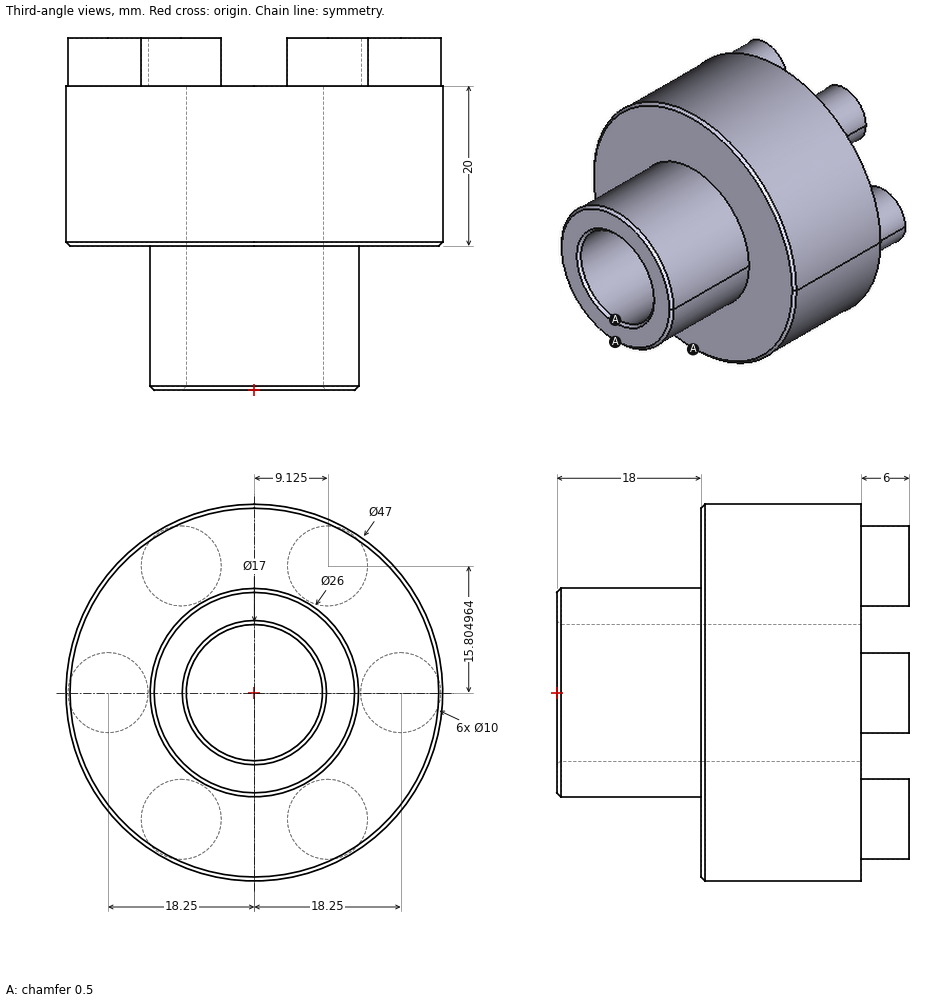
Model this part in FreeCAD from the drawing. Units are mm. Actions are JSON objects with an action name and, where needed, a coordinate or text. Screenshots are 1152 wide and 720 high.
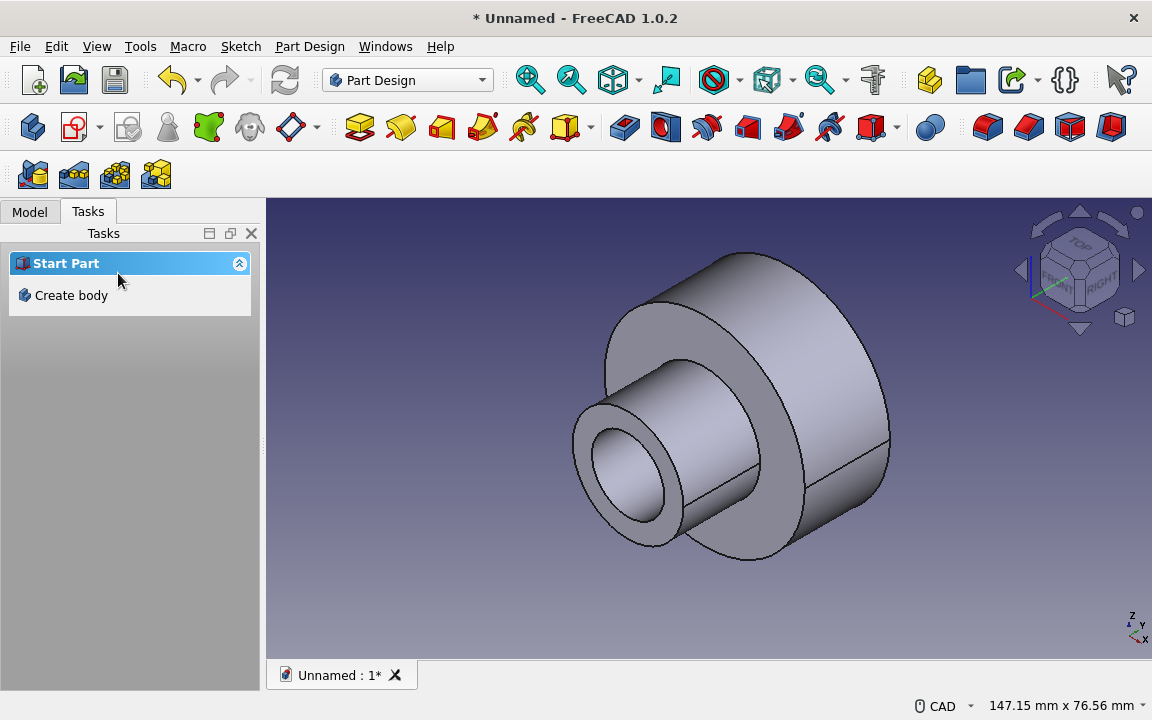
{"action": "key", "text": "4"}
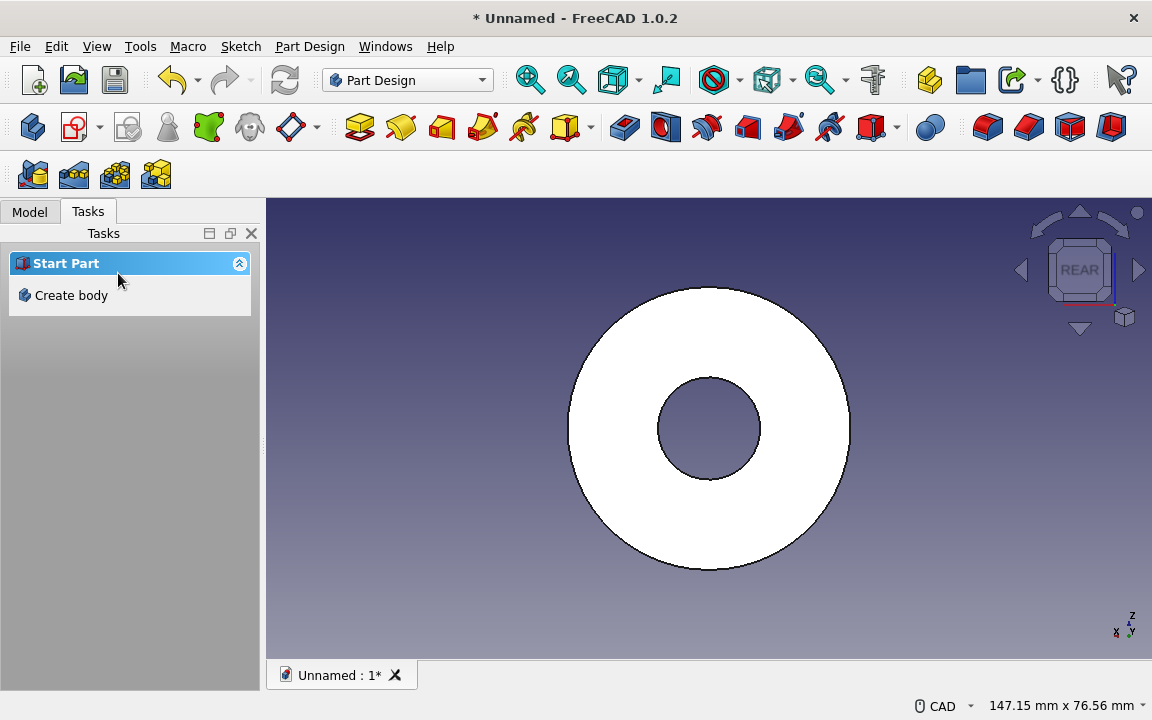
{"action": "left_click", "coordinate": [749, 347]}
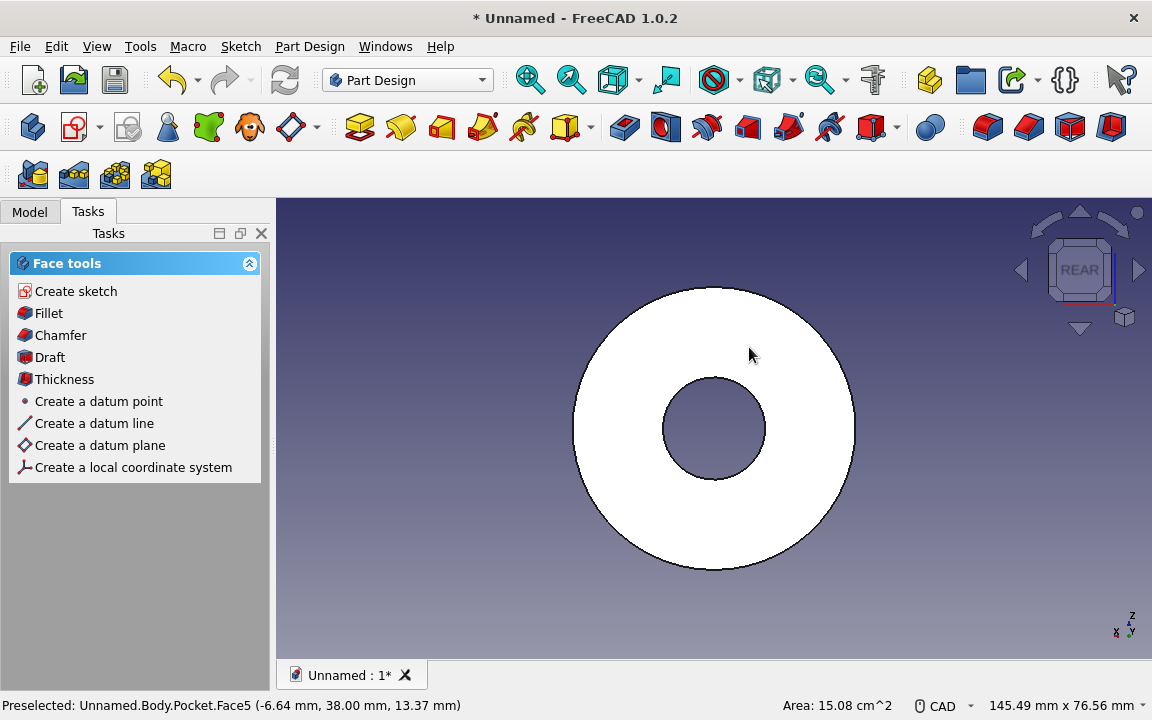
{"action": "left_click", "coordinate": [74, 128]}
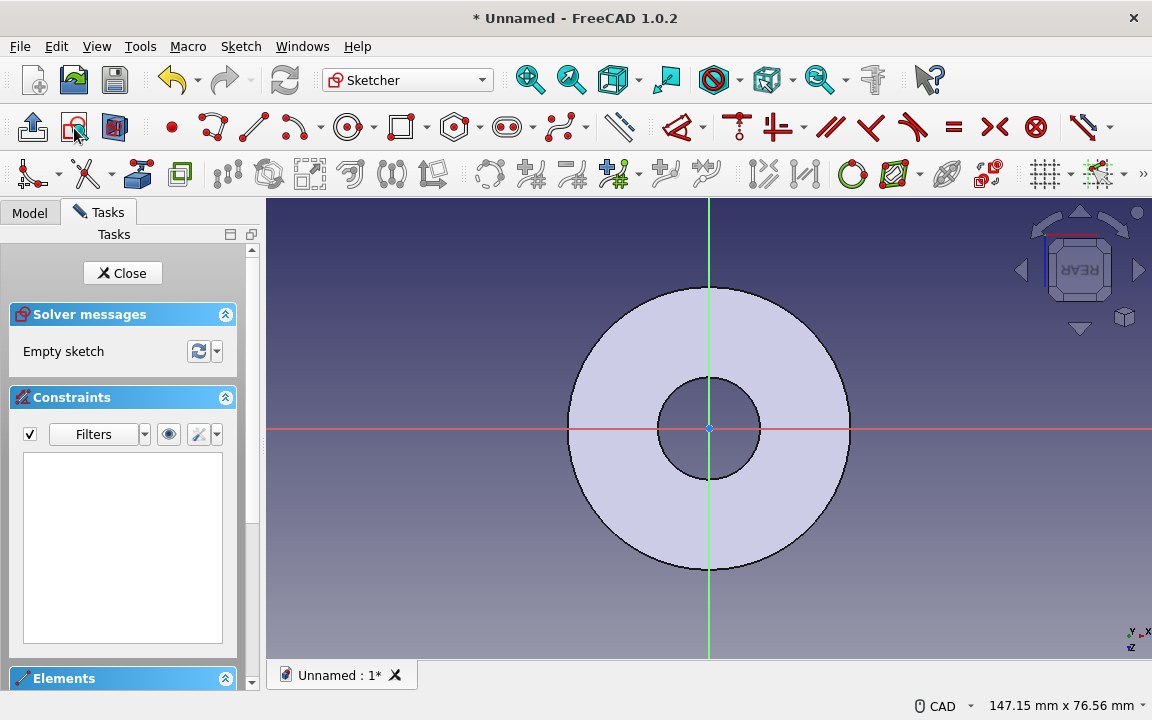
{"action": "left_click", "coordinate": [348, 128]}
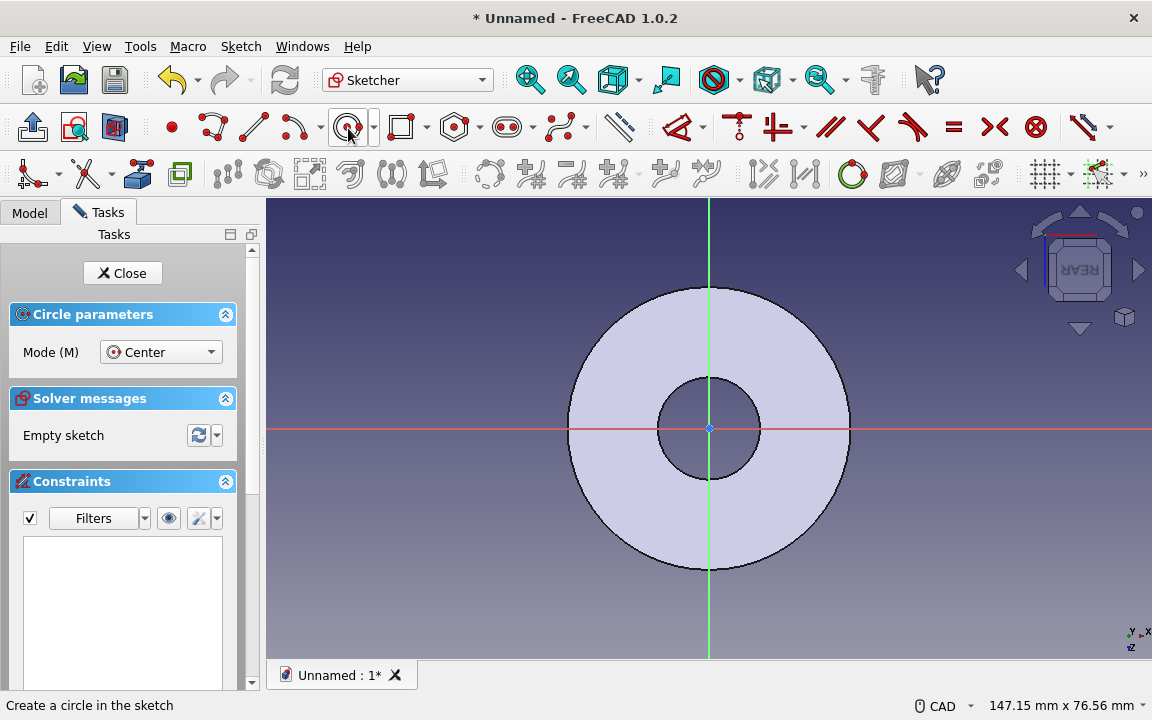
{"action": "left_click", "coordinate": [819, 429]}
{"action": "left_click", "coordinate": [840, 407]}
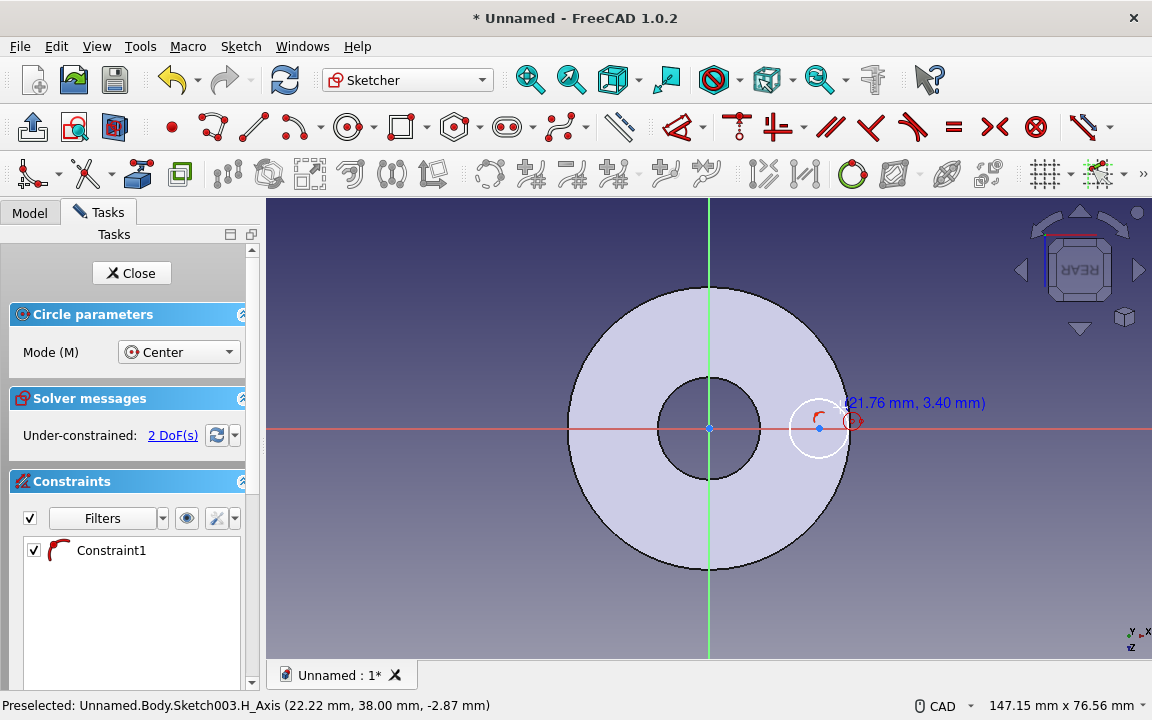
{"action": "left_click", "coordinate": [764, 524]}
{"action": "left_click", "coordinate": [785, 502]}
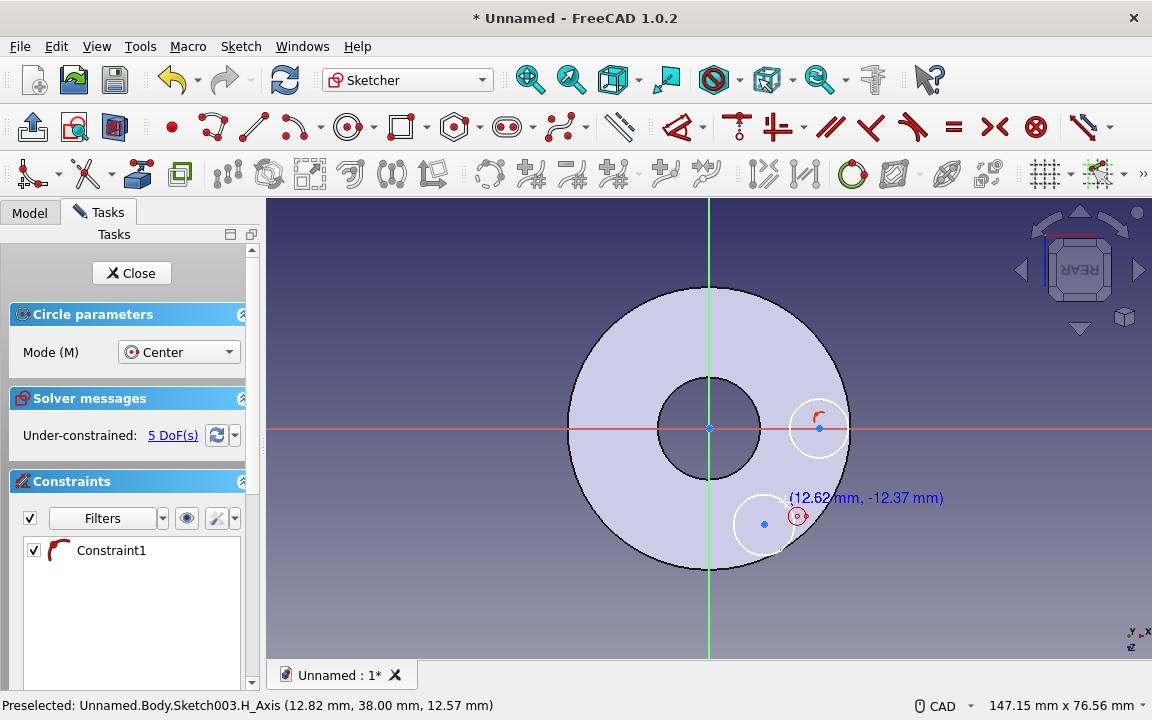
{"action": "left_click", "coordinate": [654, 524]}
{"action": "left_click", "coordinate": [675, 502]}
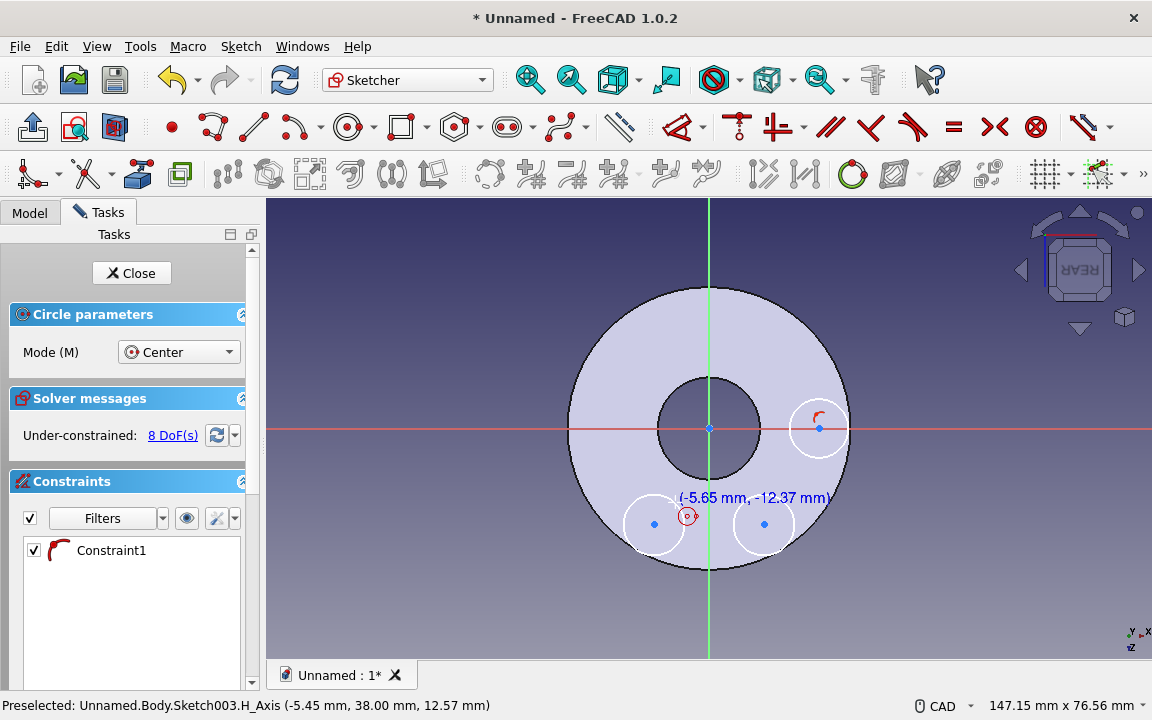
{"action": "left_click", "coordinate": [599, 429]}
{"action": "left_click", "coordinate": [620, 407]}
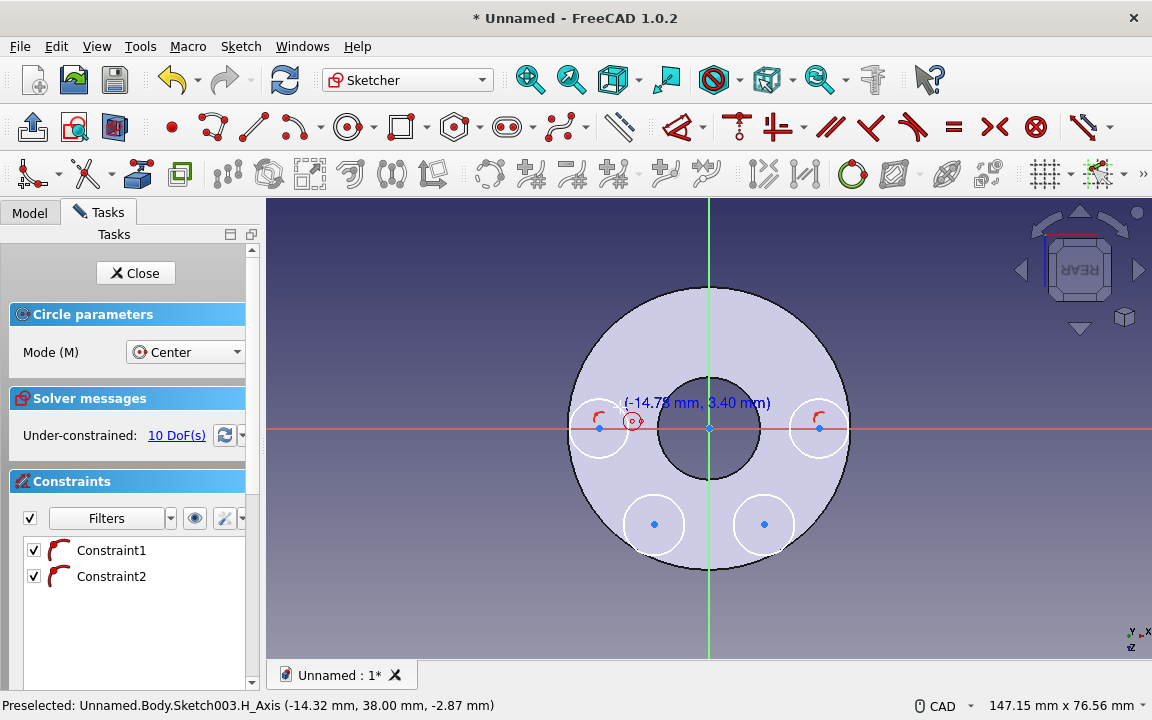
{"action": "left_click", "coordinate": [654, 333]}
{"action": "left_click", "coordinate": [675, 312]}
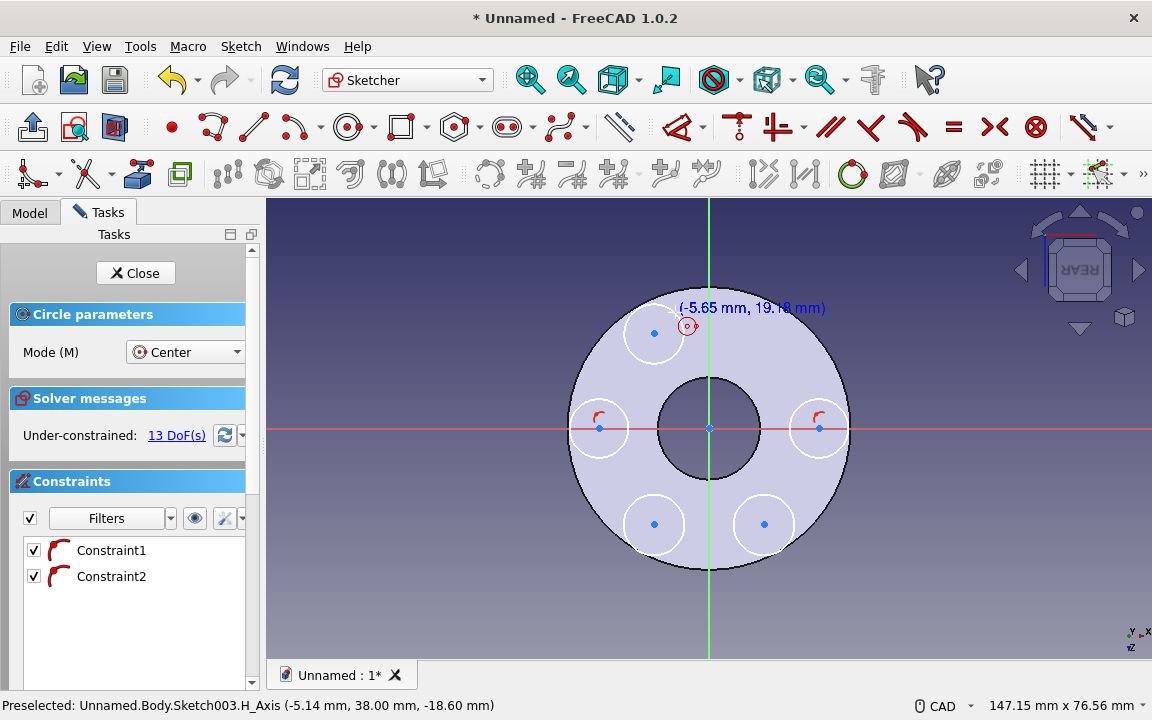
{"action": "left_click", "coordinate": [764, 333]}
{"action": "left_click", "coordinate": [785, 312]}
{"action": "key", "text": "Escape"}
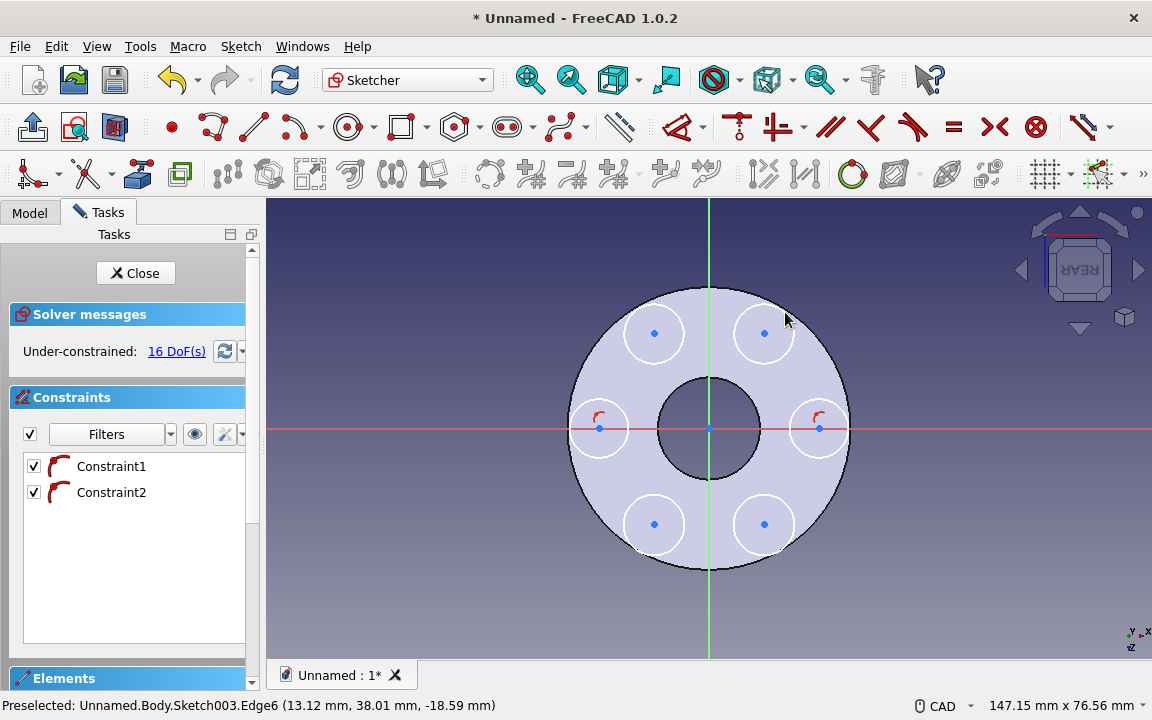
{"action": "left_click", "coordinate": [840, 408]}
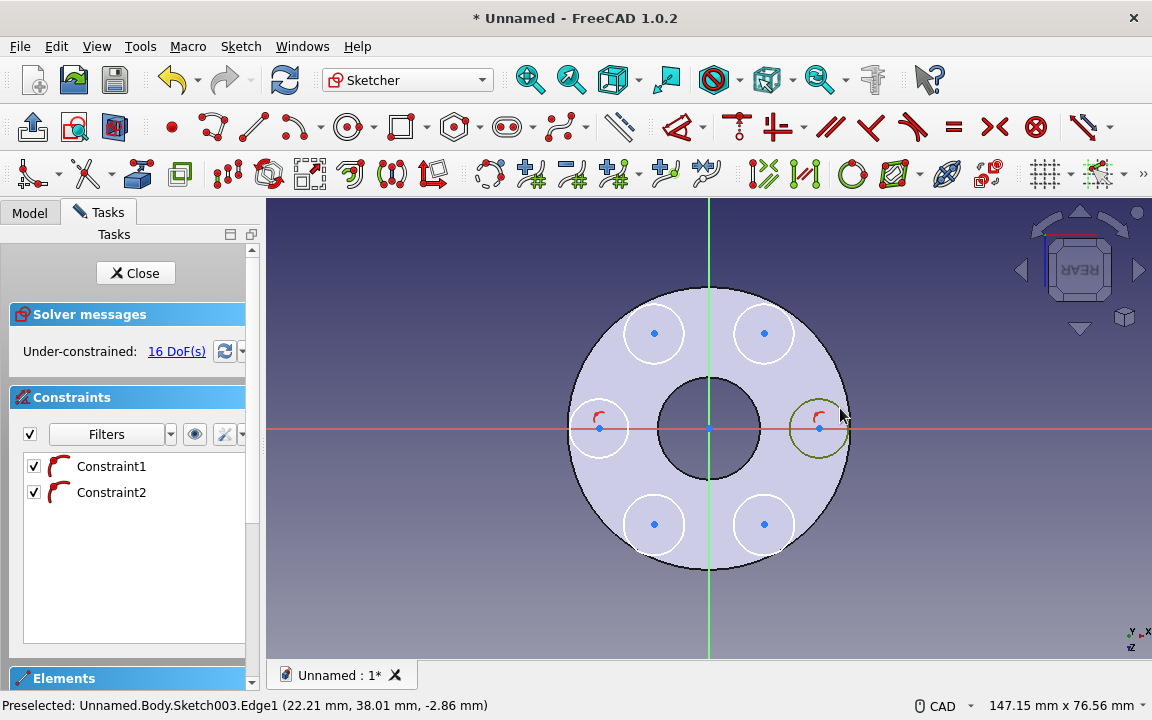
{"action": "left_click", "coordinate": [785, 503]}